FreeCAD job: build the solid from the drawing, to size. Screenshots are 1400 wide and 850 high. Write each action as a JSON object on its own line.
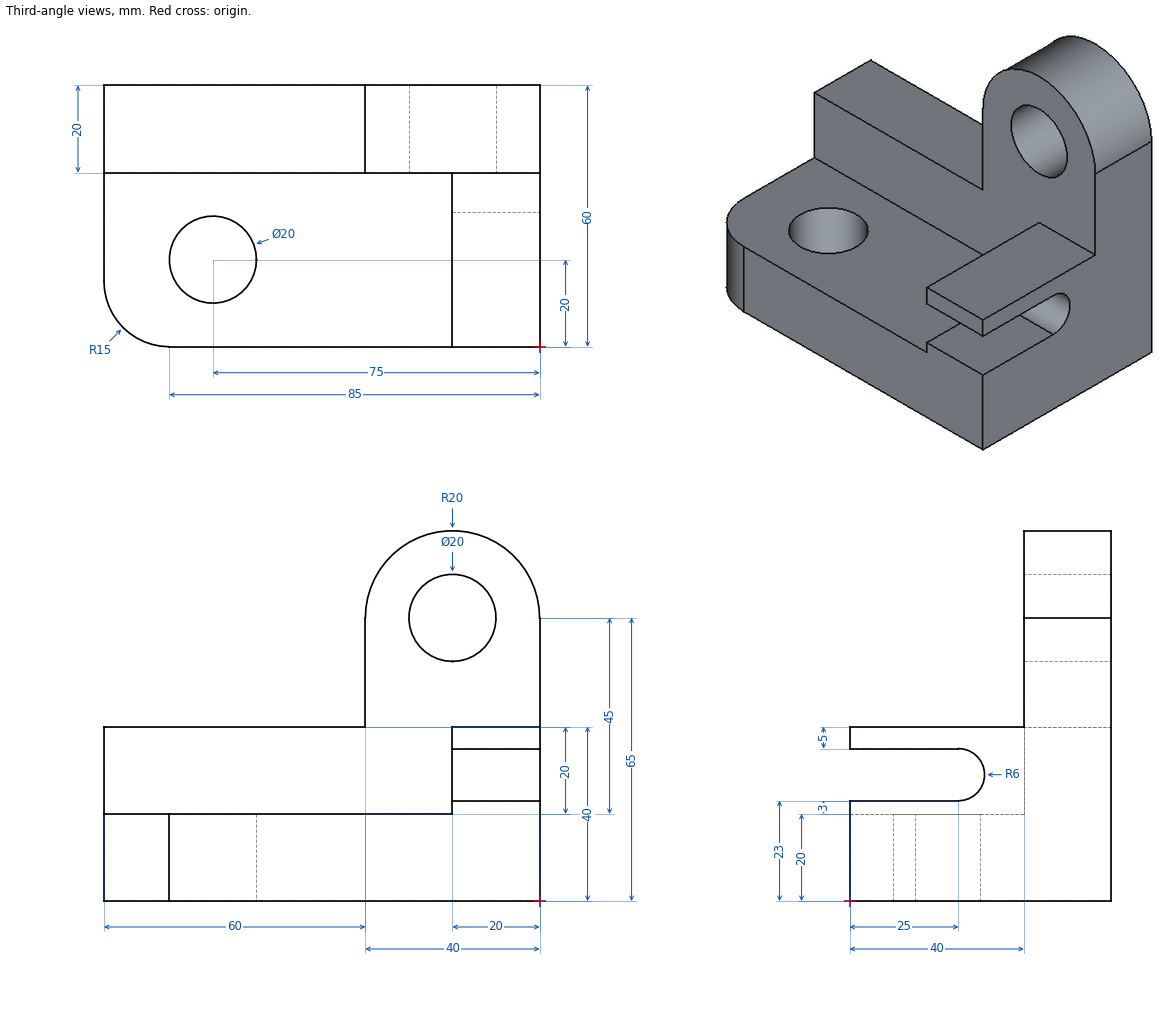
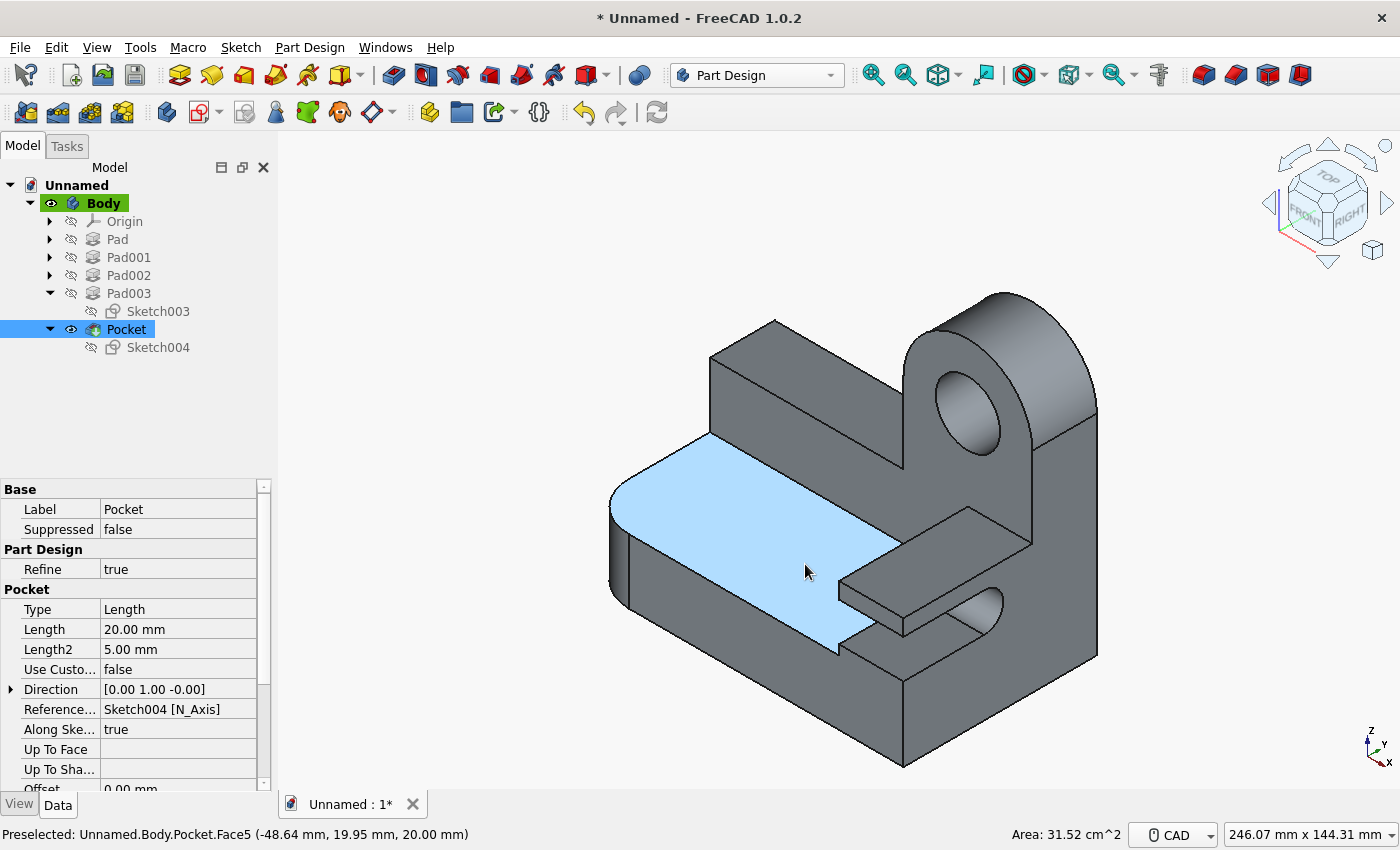
{"action": "left_click", "coordinate": [200, 112]}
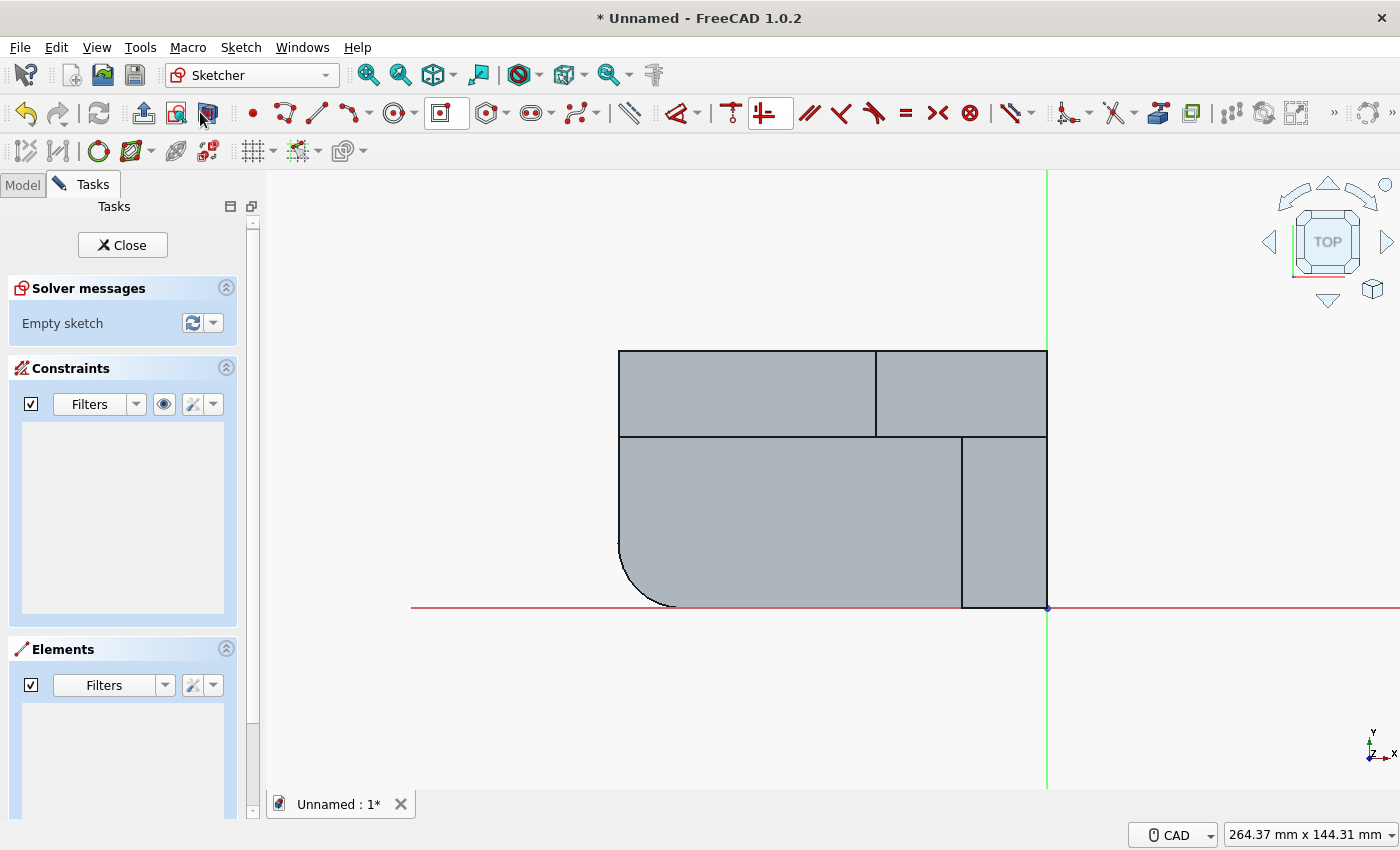
{"action": "key", "text": "q s"}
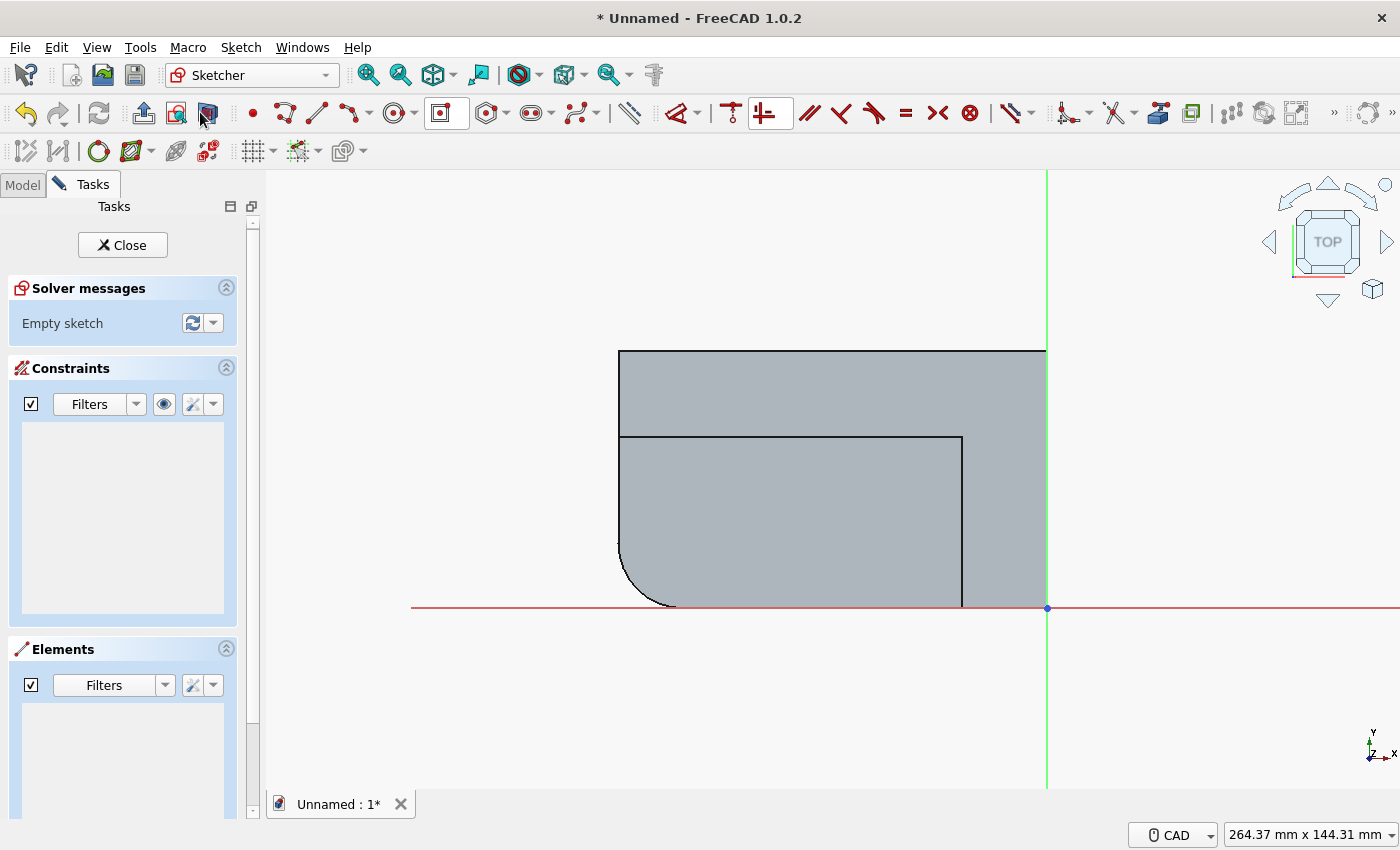
{"action": "scroll", "coordinate": [716, 533], "scroll_direction": "up", "scroll_amount": 8}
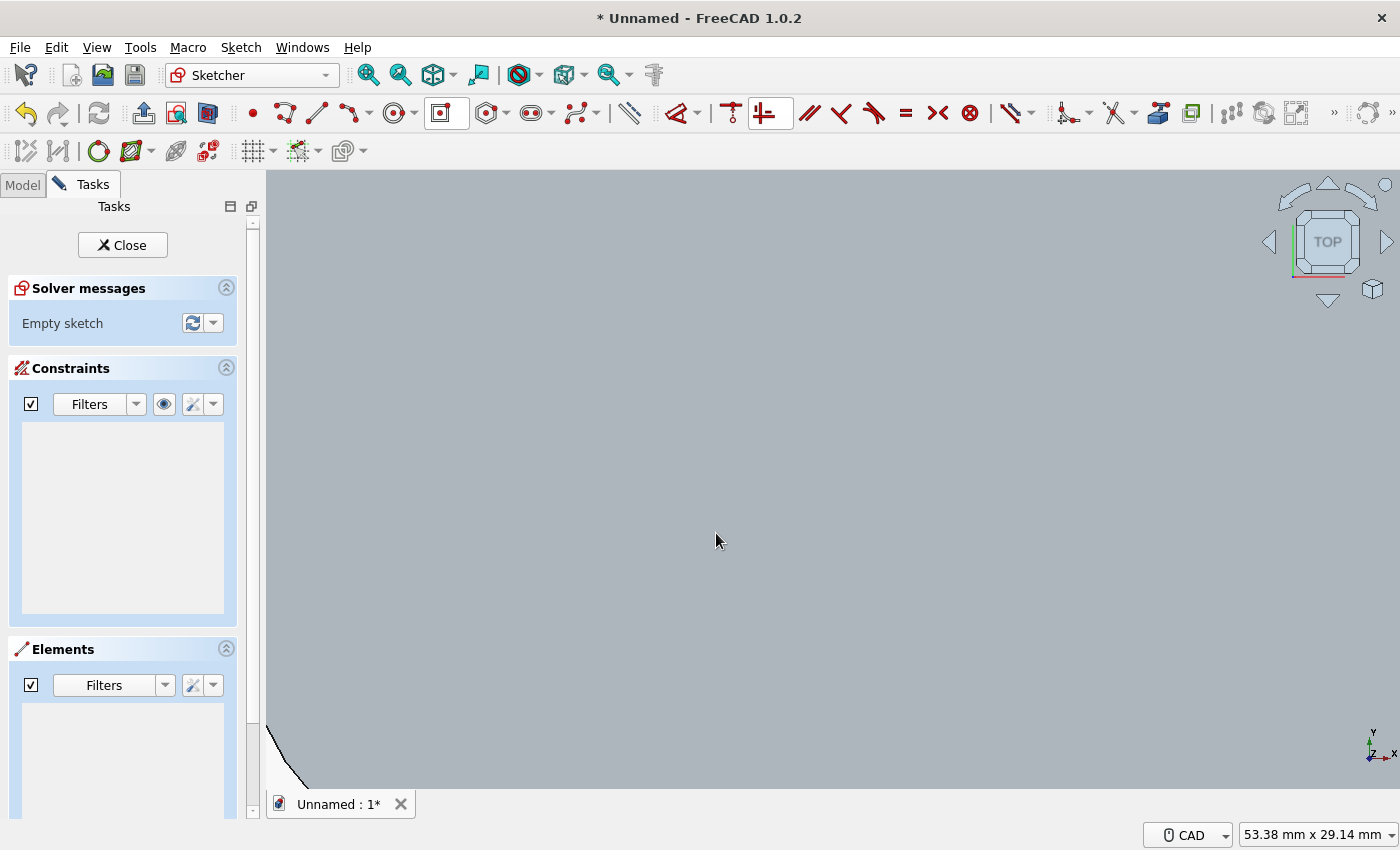
{"action": "key", "text": "g c"}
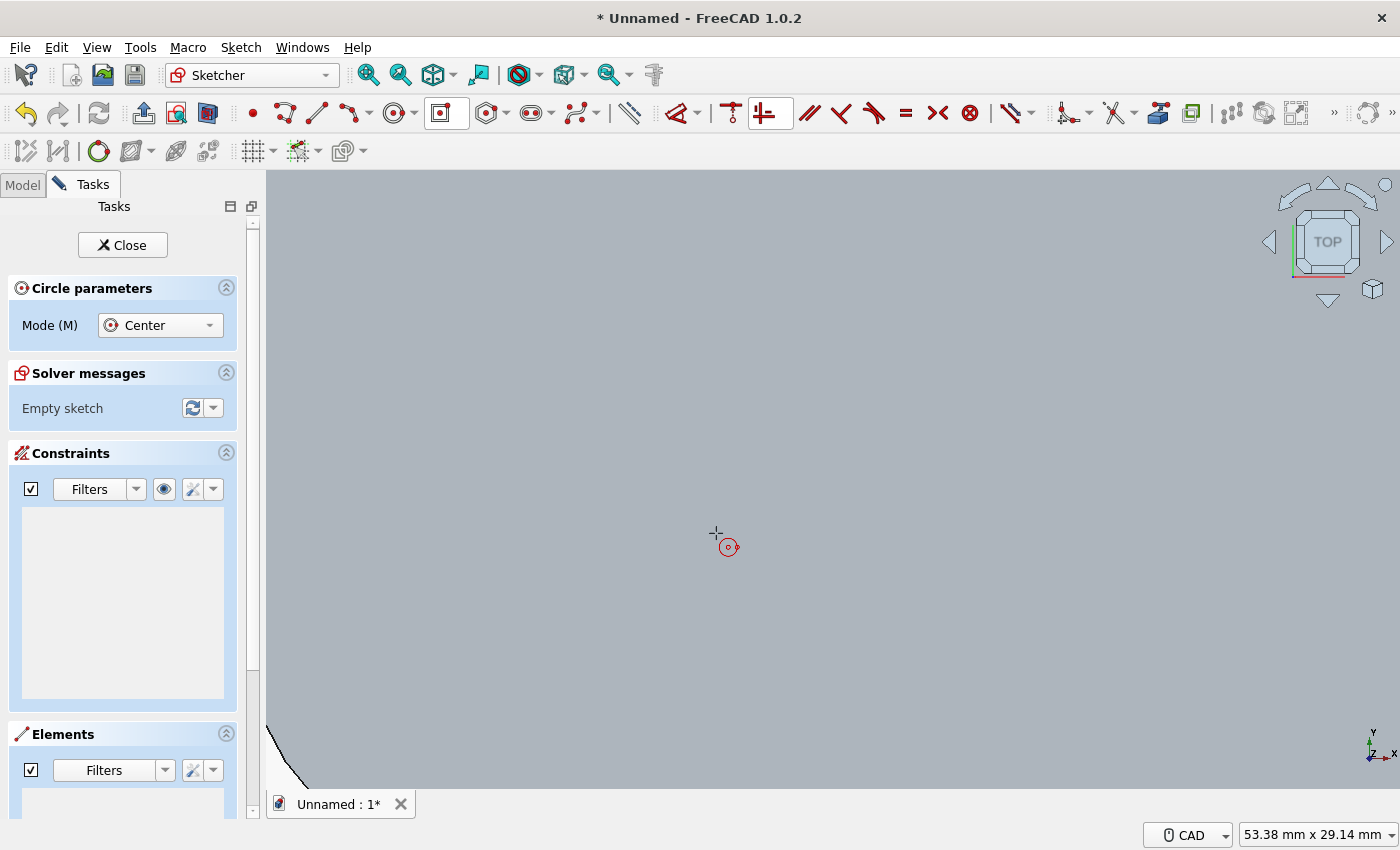
{"action": "left_click", "coordinate": [763, 478]}
{"action": "left_click", "coordinate": [913, 328]}
{"action": "key", "text": "Escape"}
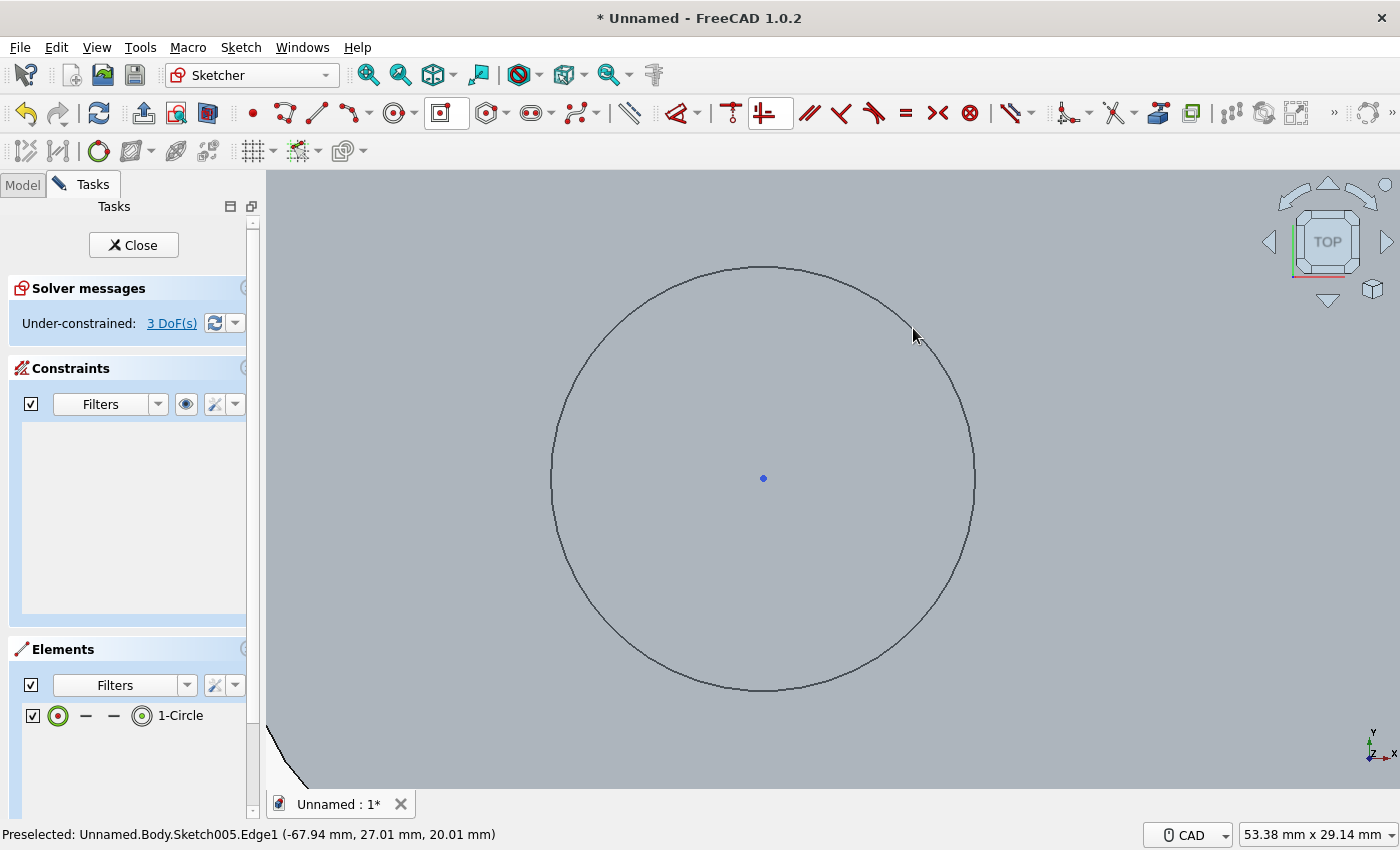
{"action": "key", "text": "d"}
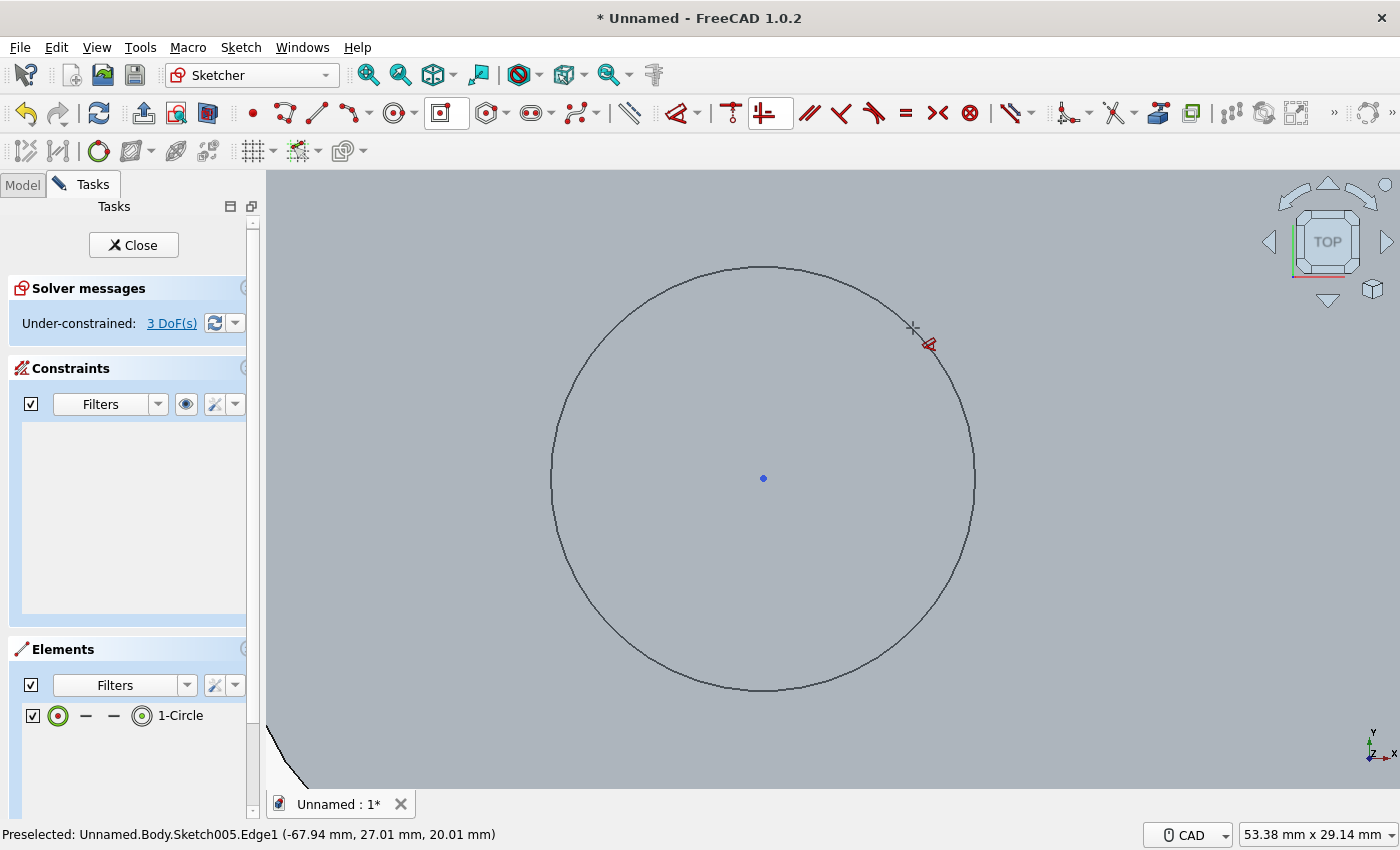
{"action": "left_click", "coordinate": [913, 329]}
{"action": "left_click", "coordinate": [936, 306]}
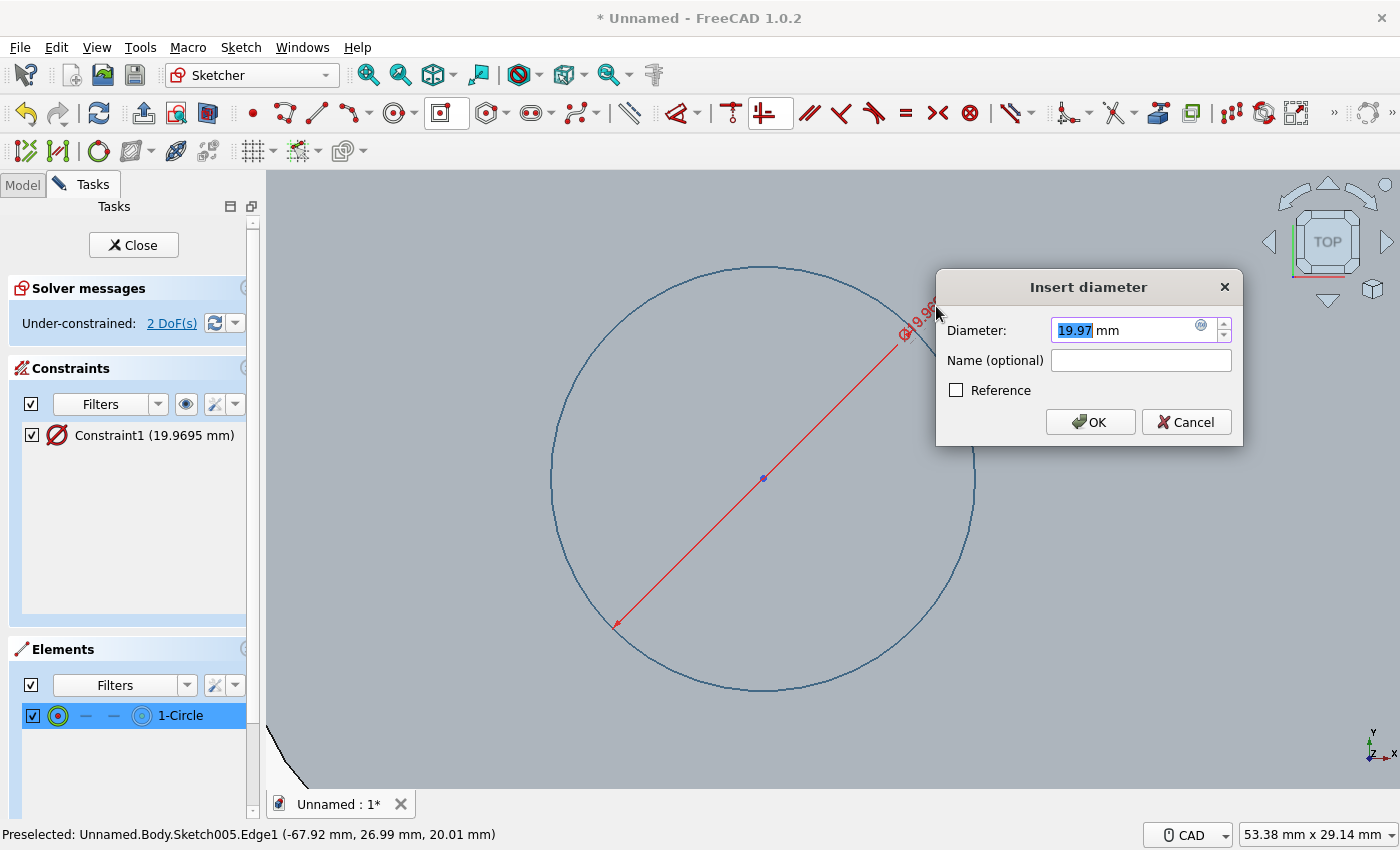
{"action": "type", "text": "20"}
{"action": "key", "text": "Return"}